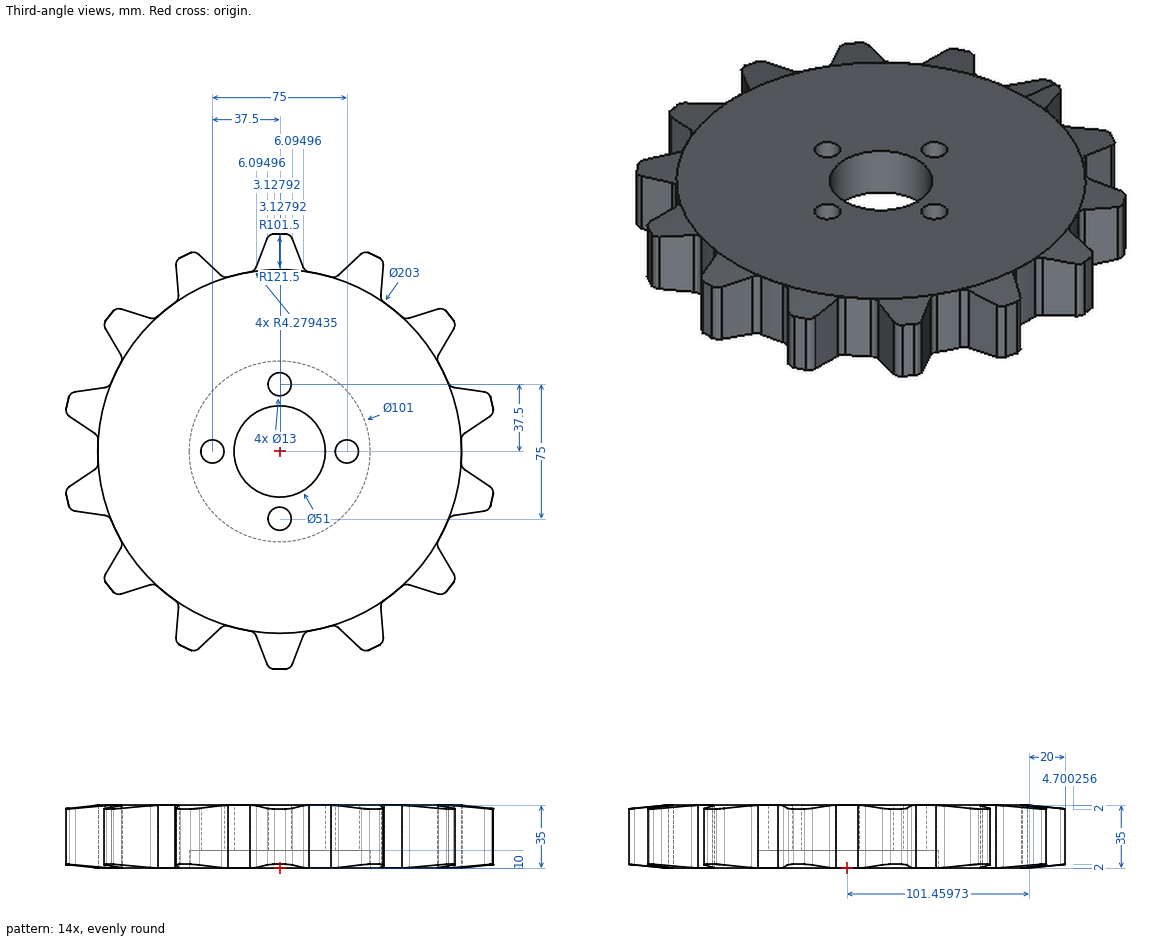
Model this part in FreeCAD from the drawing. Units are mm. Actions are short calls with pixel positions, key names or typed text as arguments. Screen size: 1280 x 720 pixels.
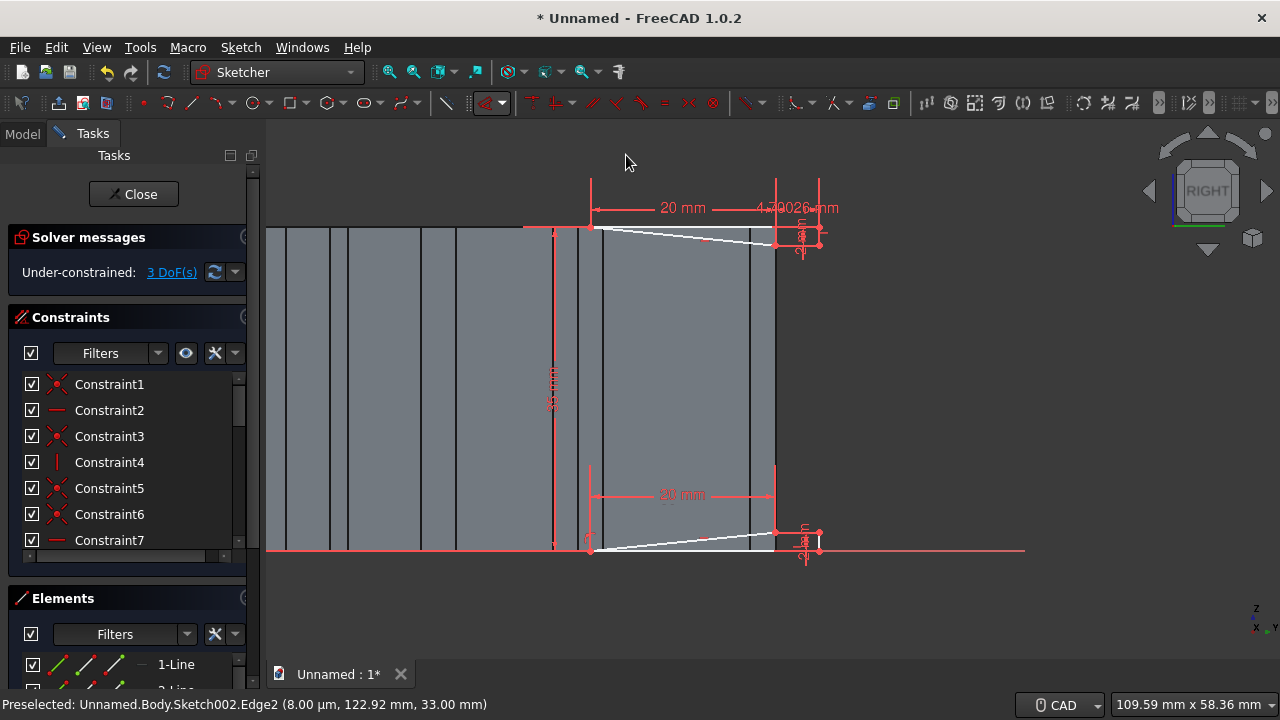
click(789, 533)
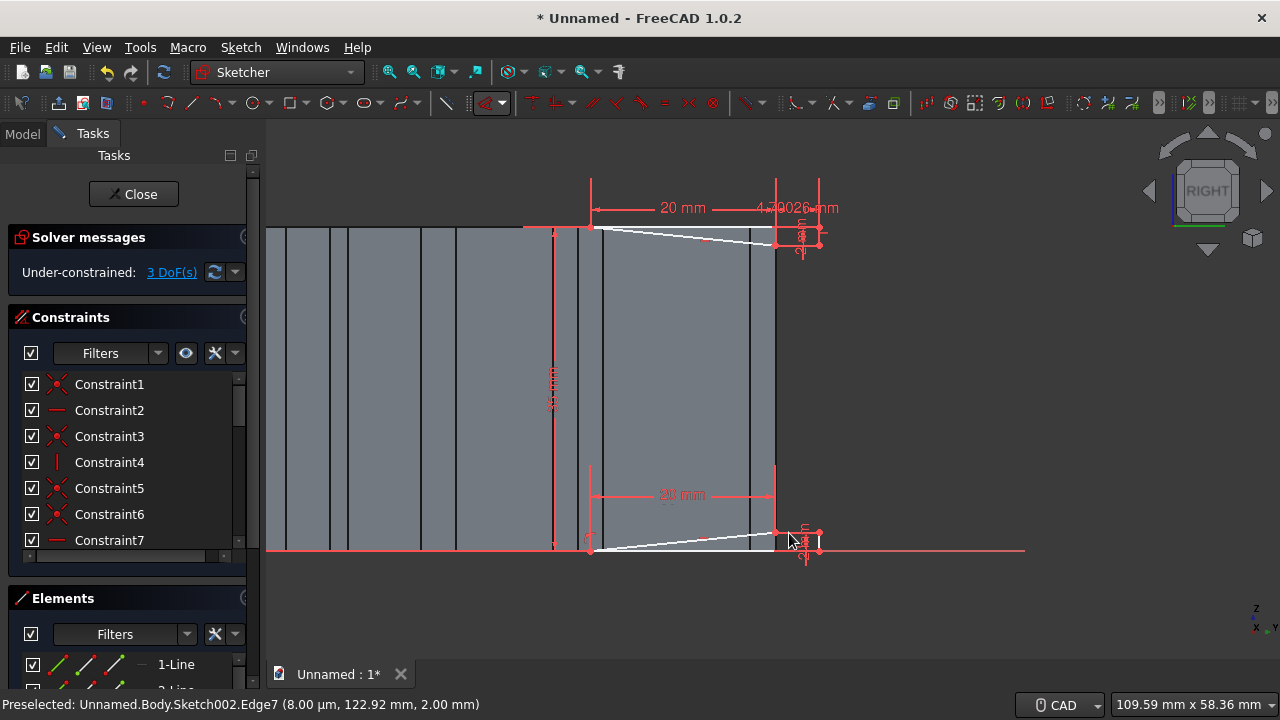
click(504, 104)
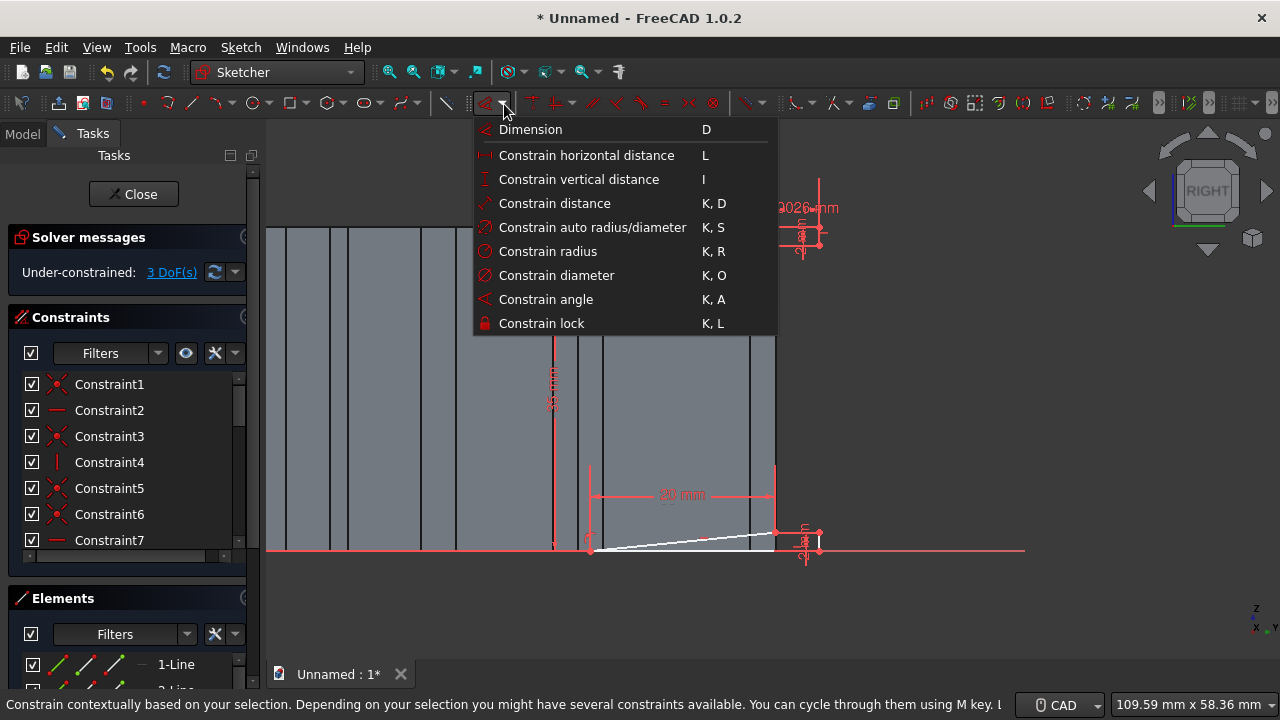
click(626, 155)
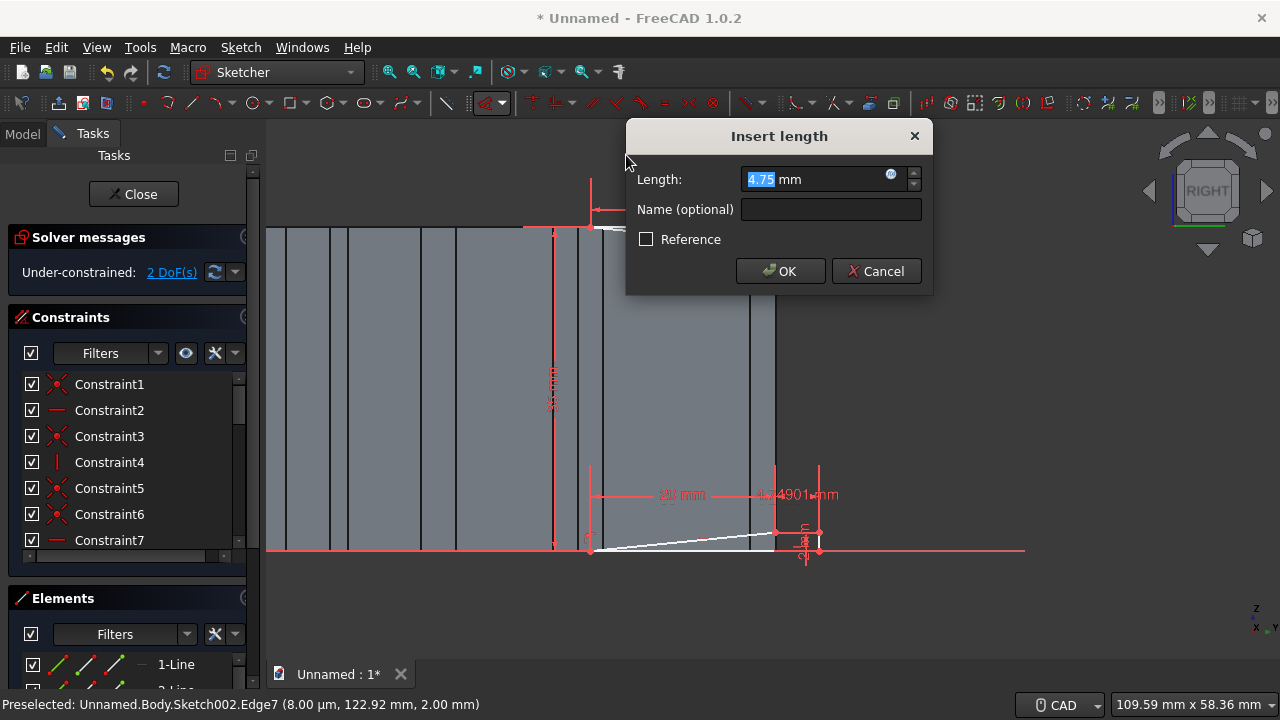
text(4.700256)
key(Return)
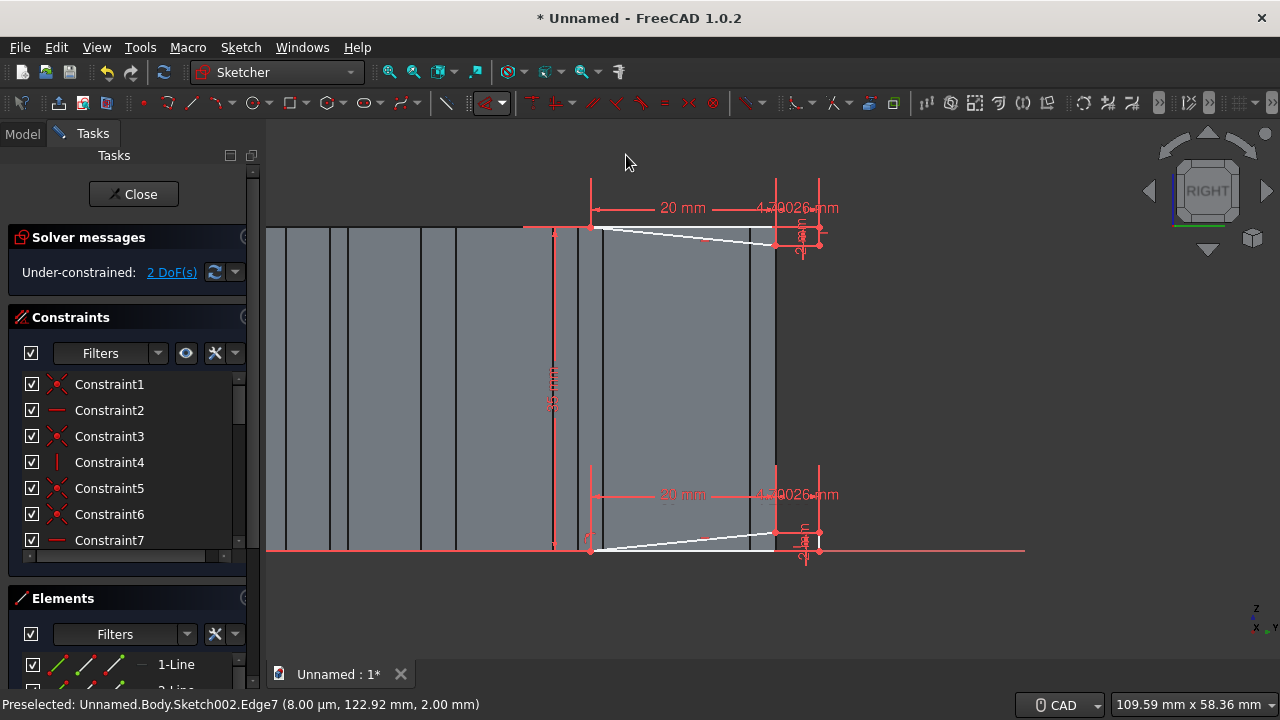
click(591, 227)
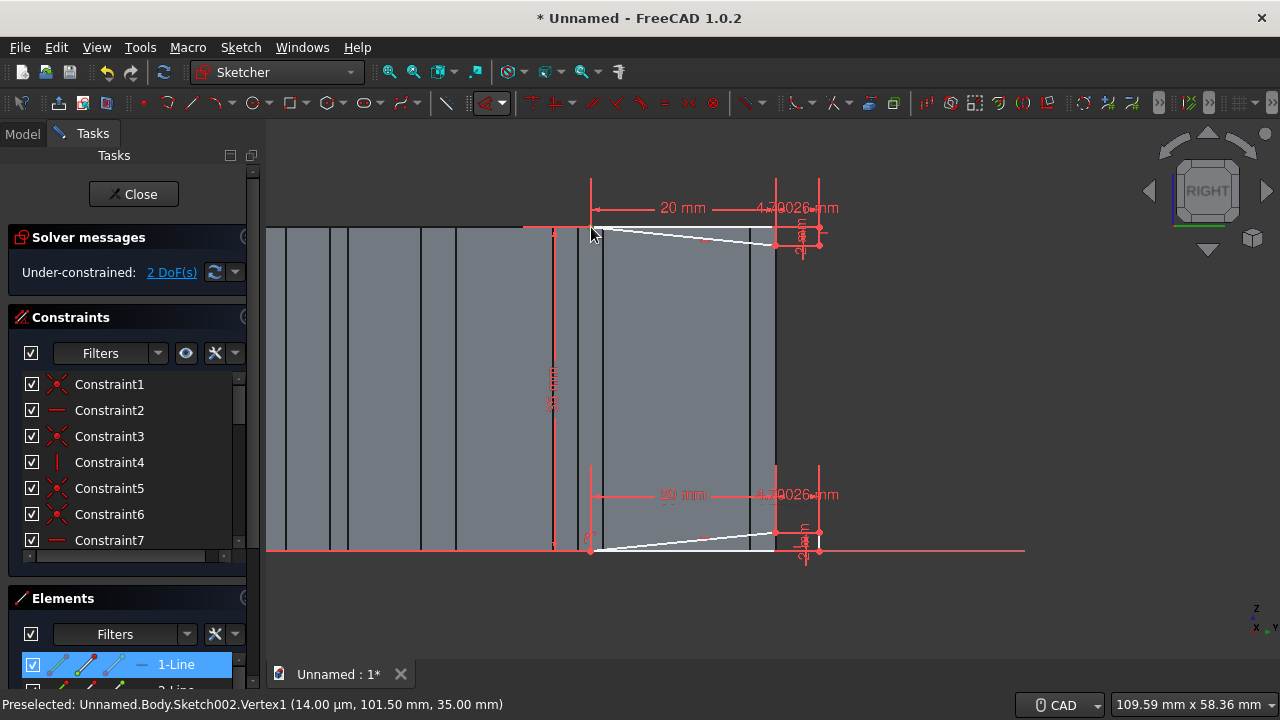
click(504, 104)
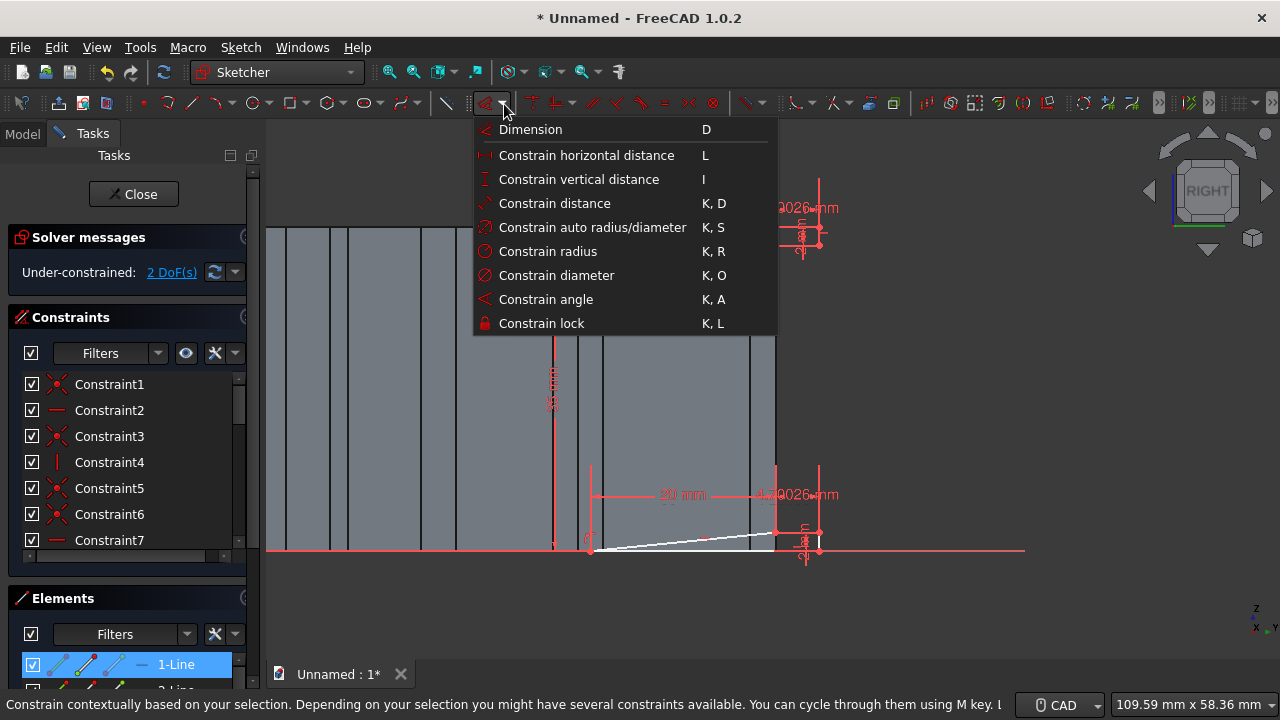
click(626, 155)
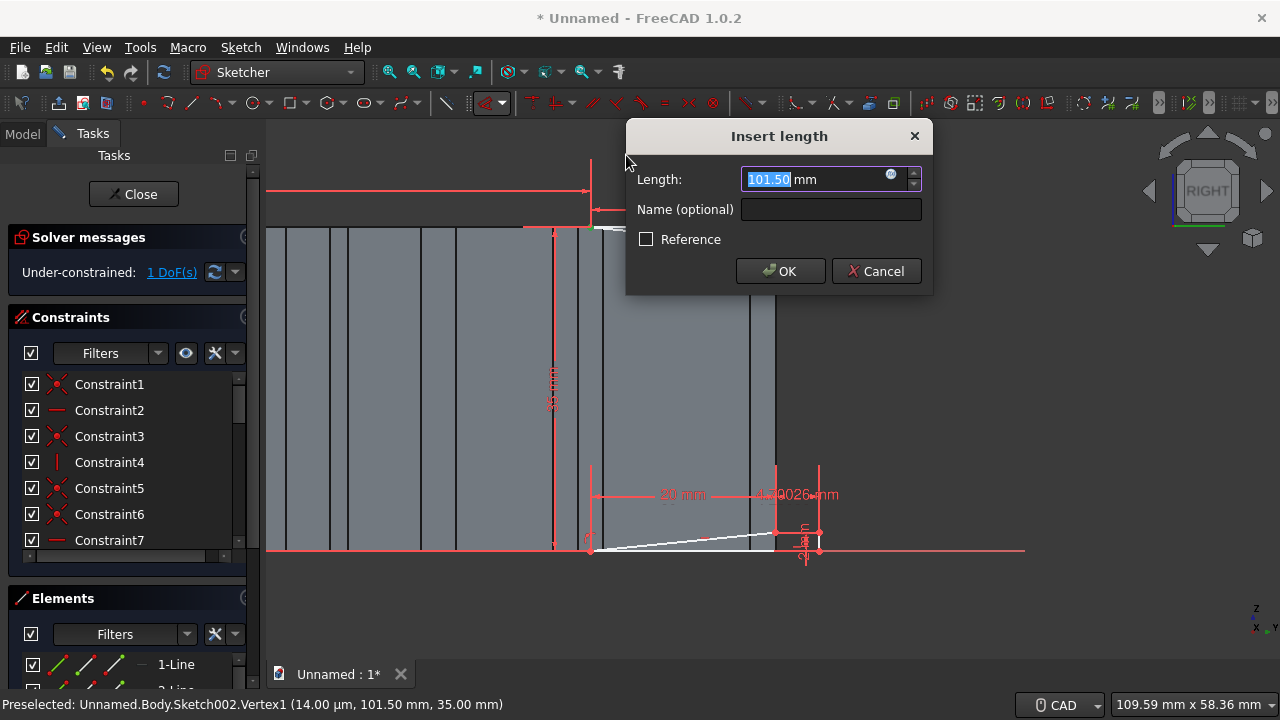
text(101.45973)
key(Return)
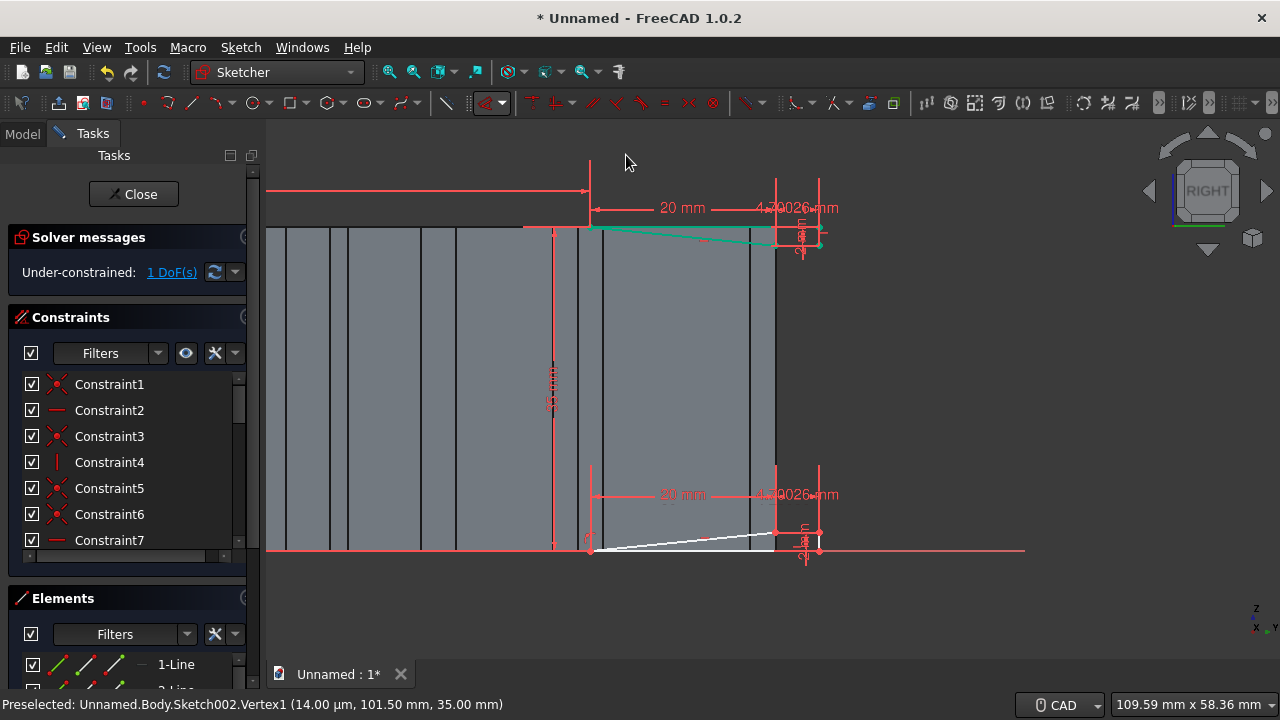
click(591, 551)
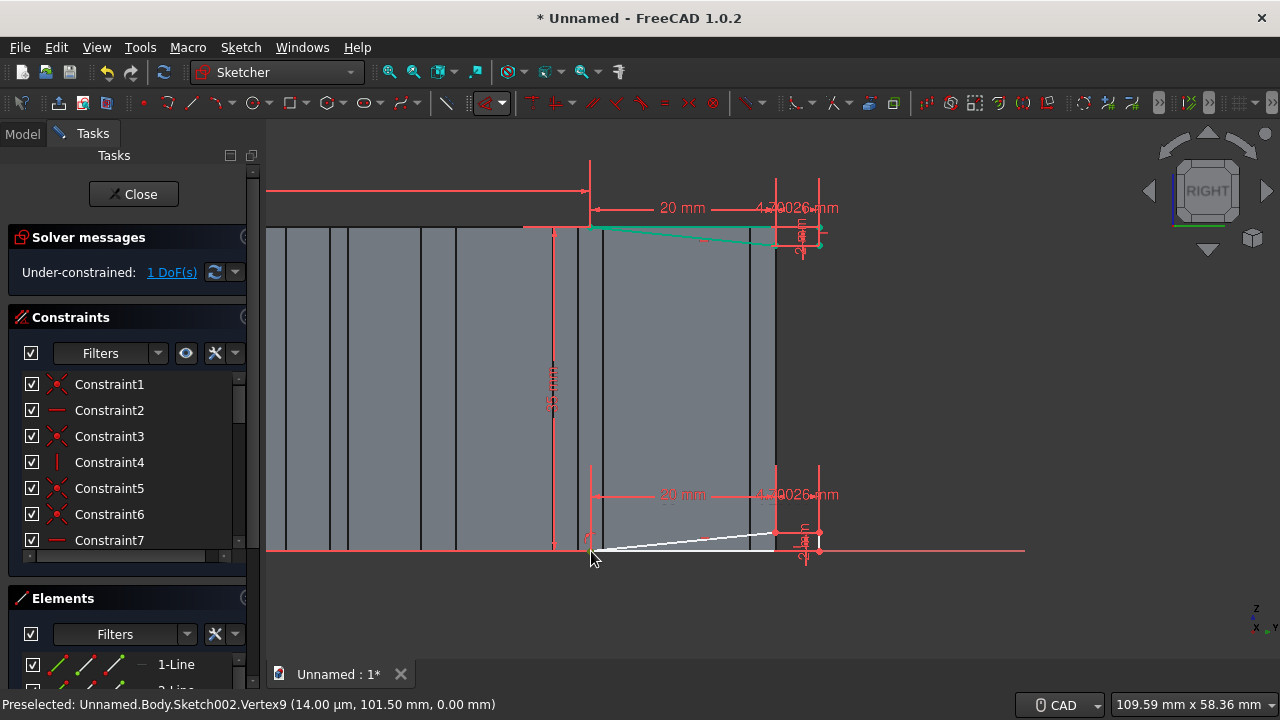
key(l)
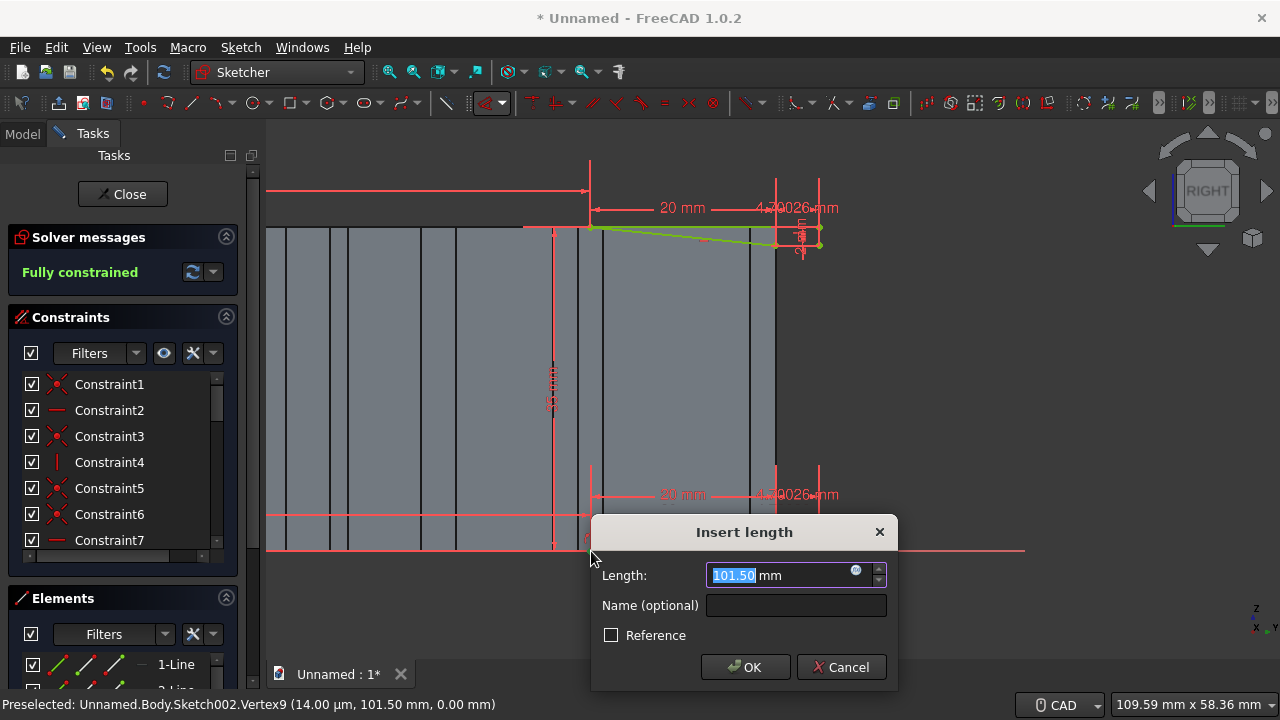
text(101.45973)
key(Return)